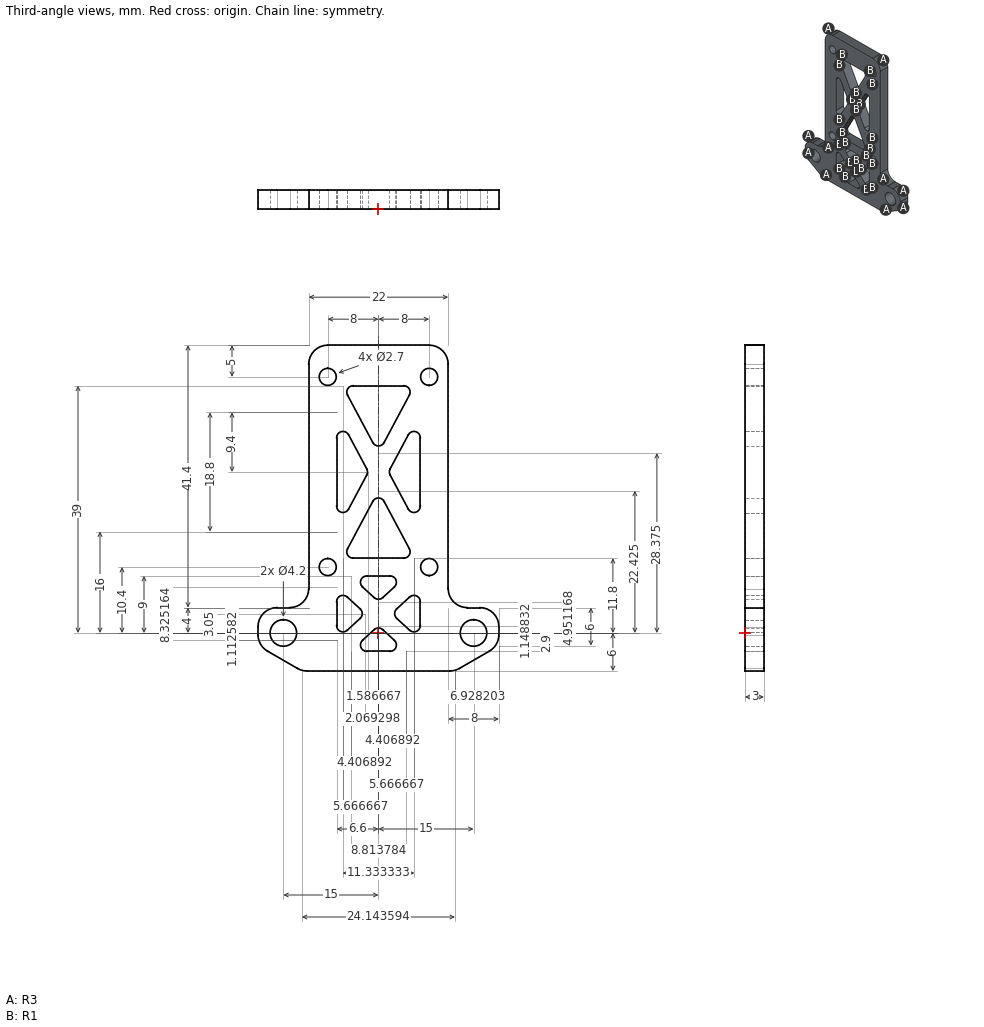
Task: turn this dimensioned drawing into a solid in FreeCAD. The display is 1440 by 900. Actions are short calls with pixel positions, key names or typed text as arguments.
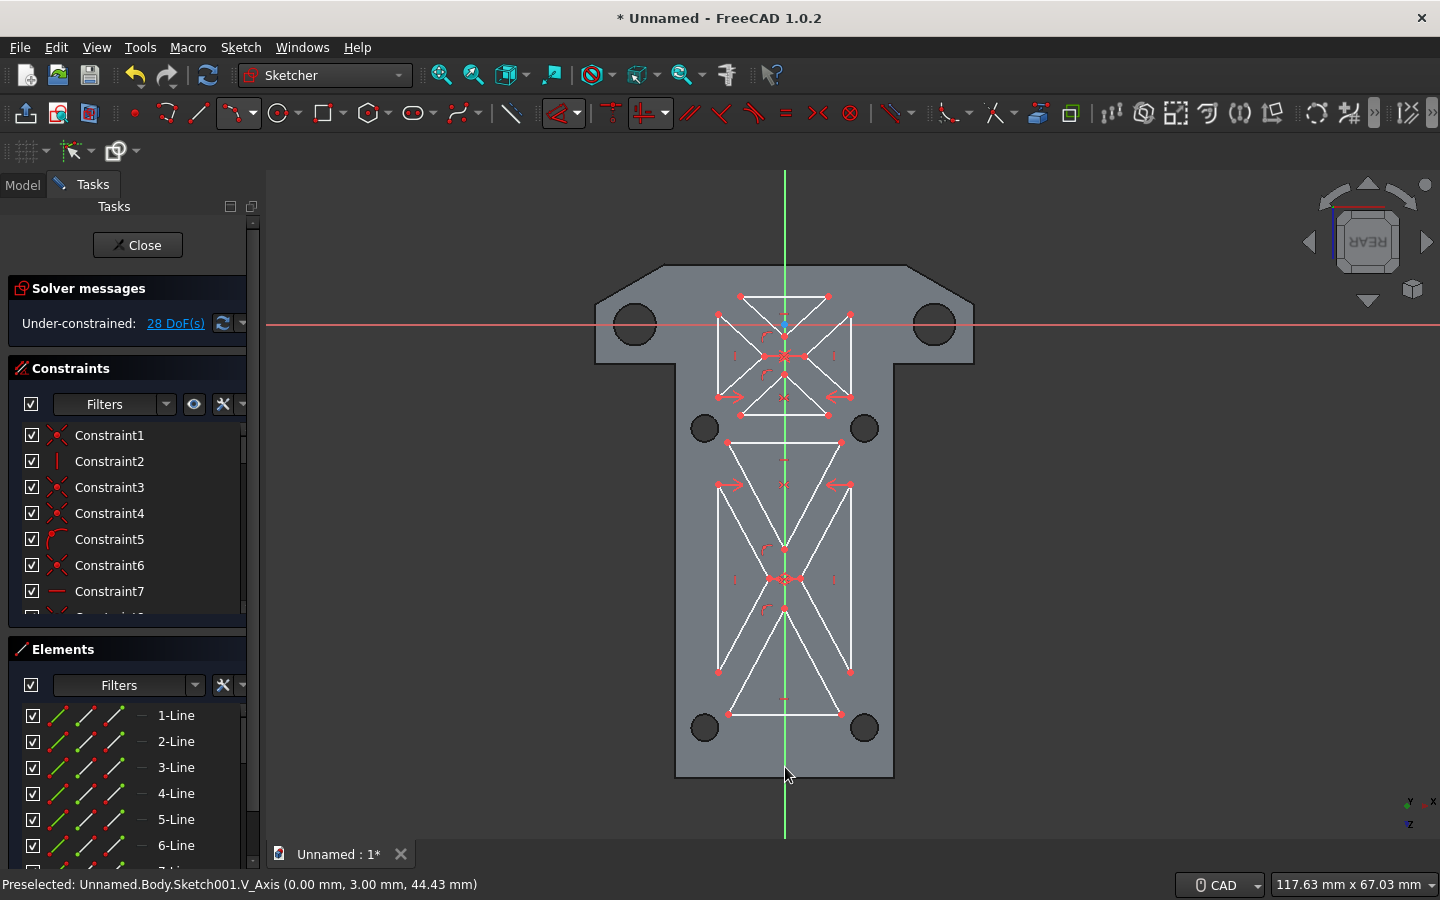
click(558, 114)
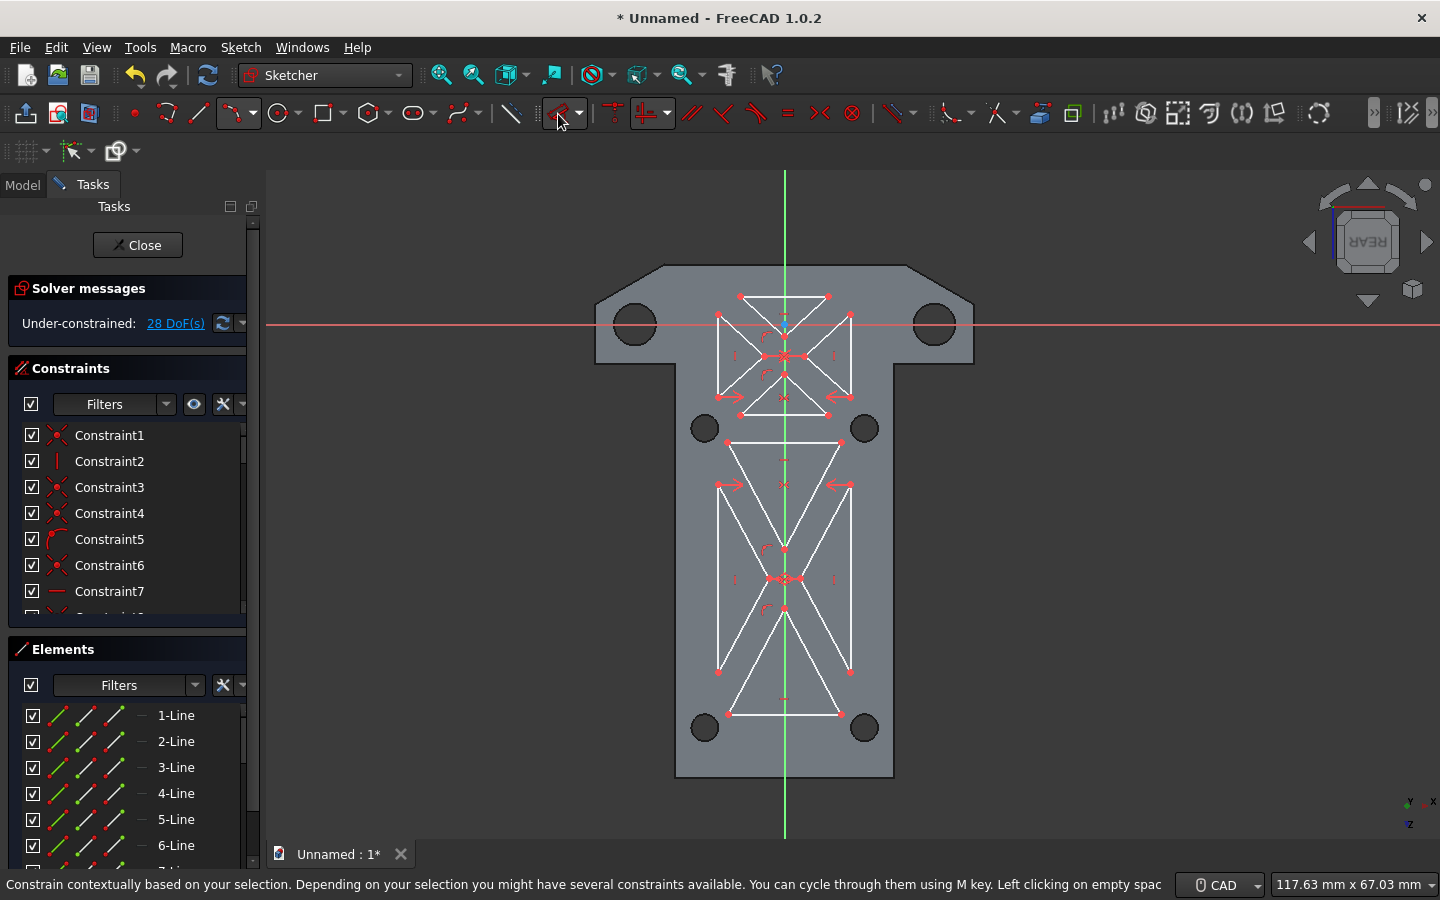
click(741, 415)
click(683, 370)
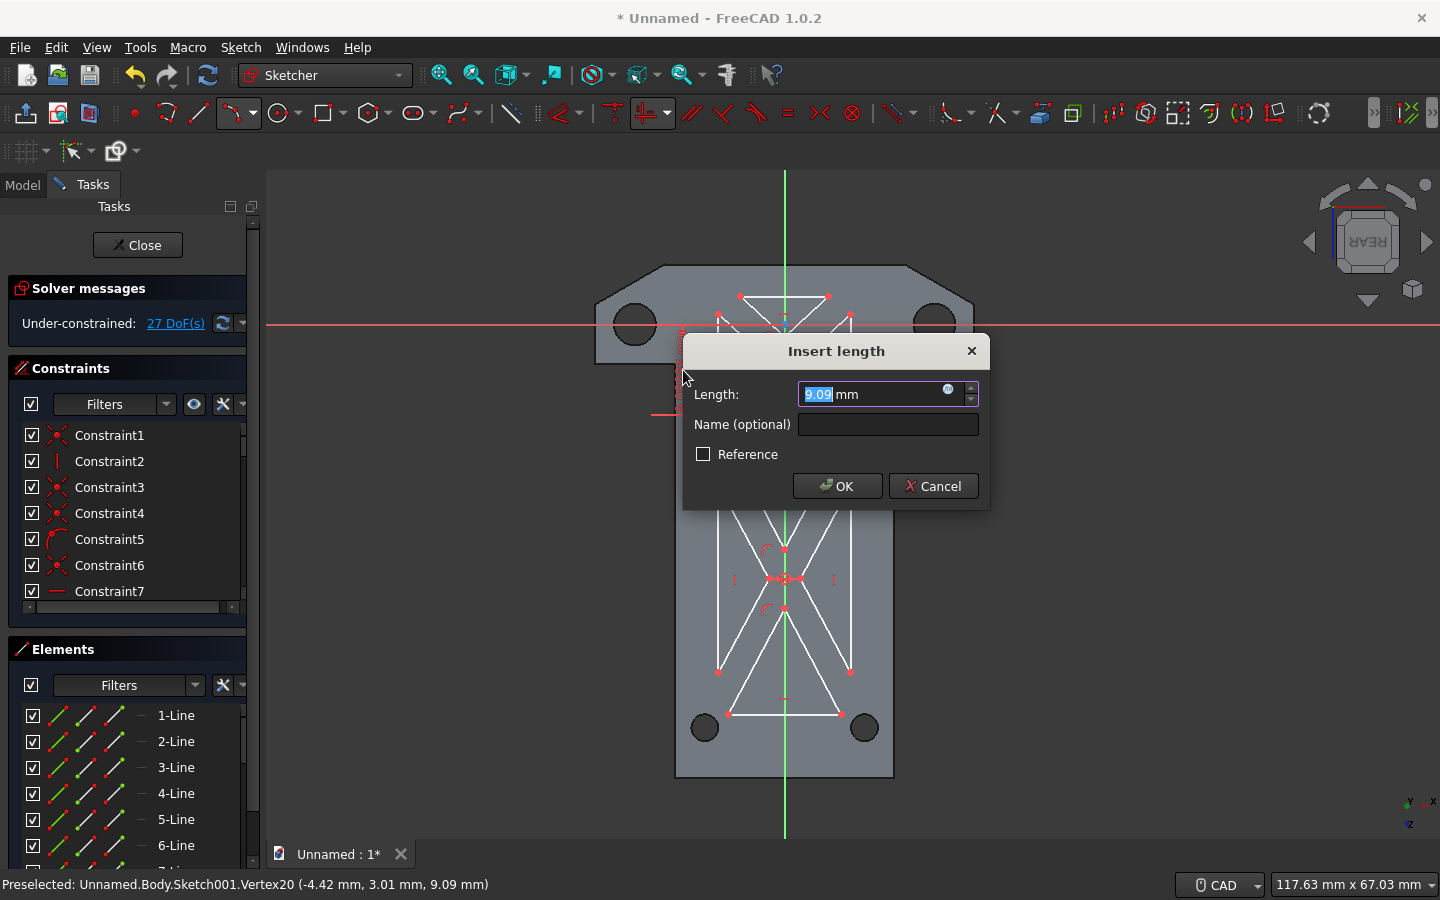
text(9)
key(Return)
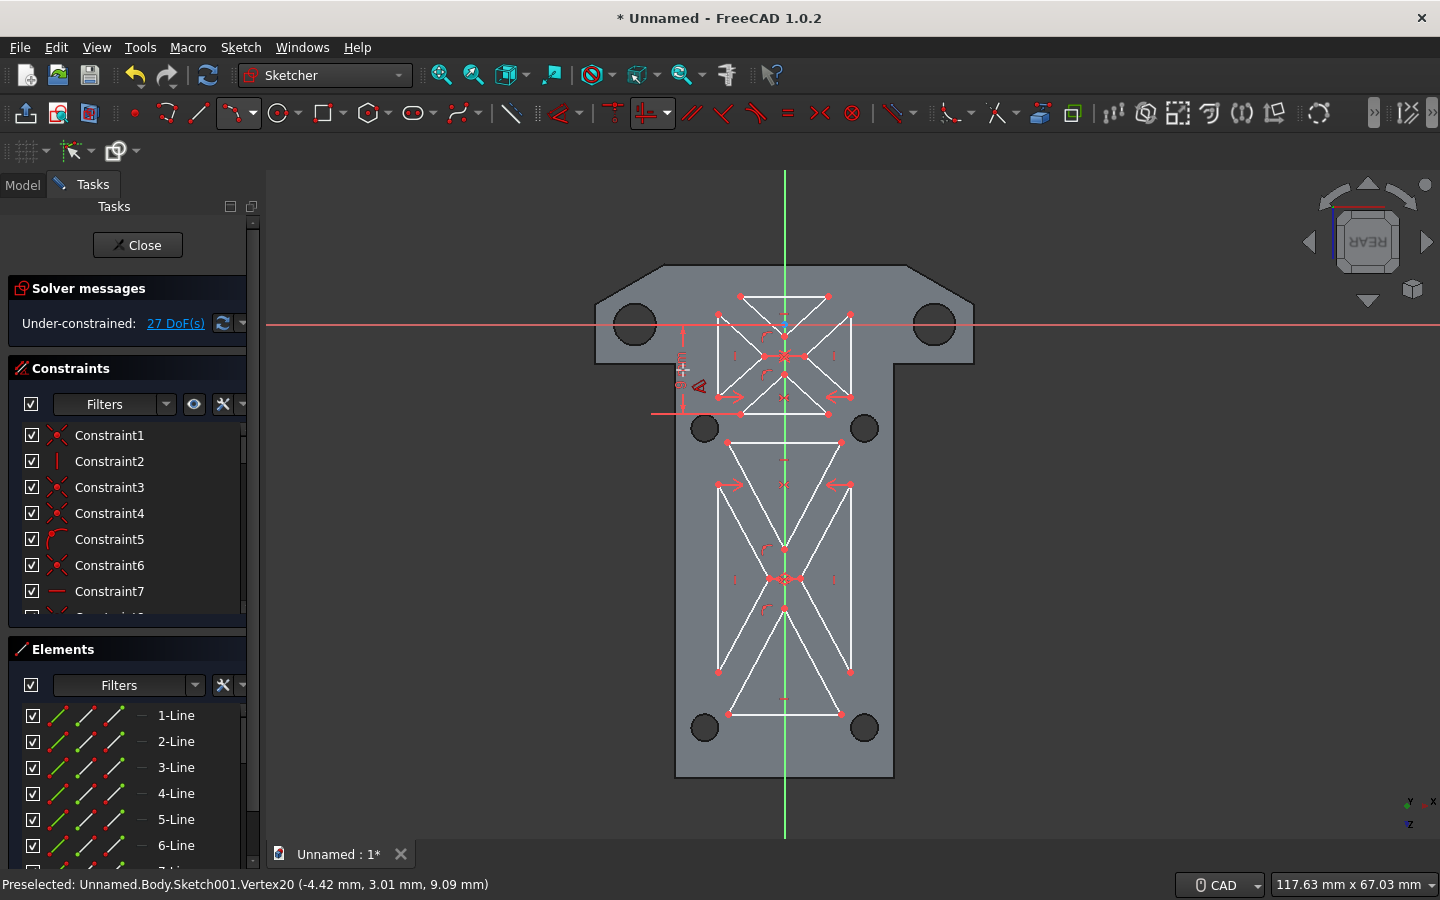
click(718, 485)
click(684, 405)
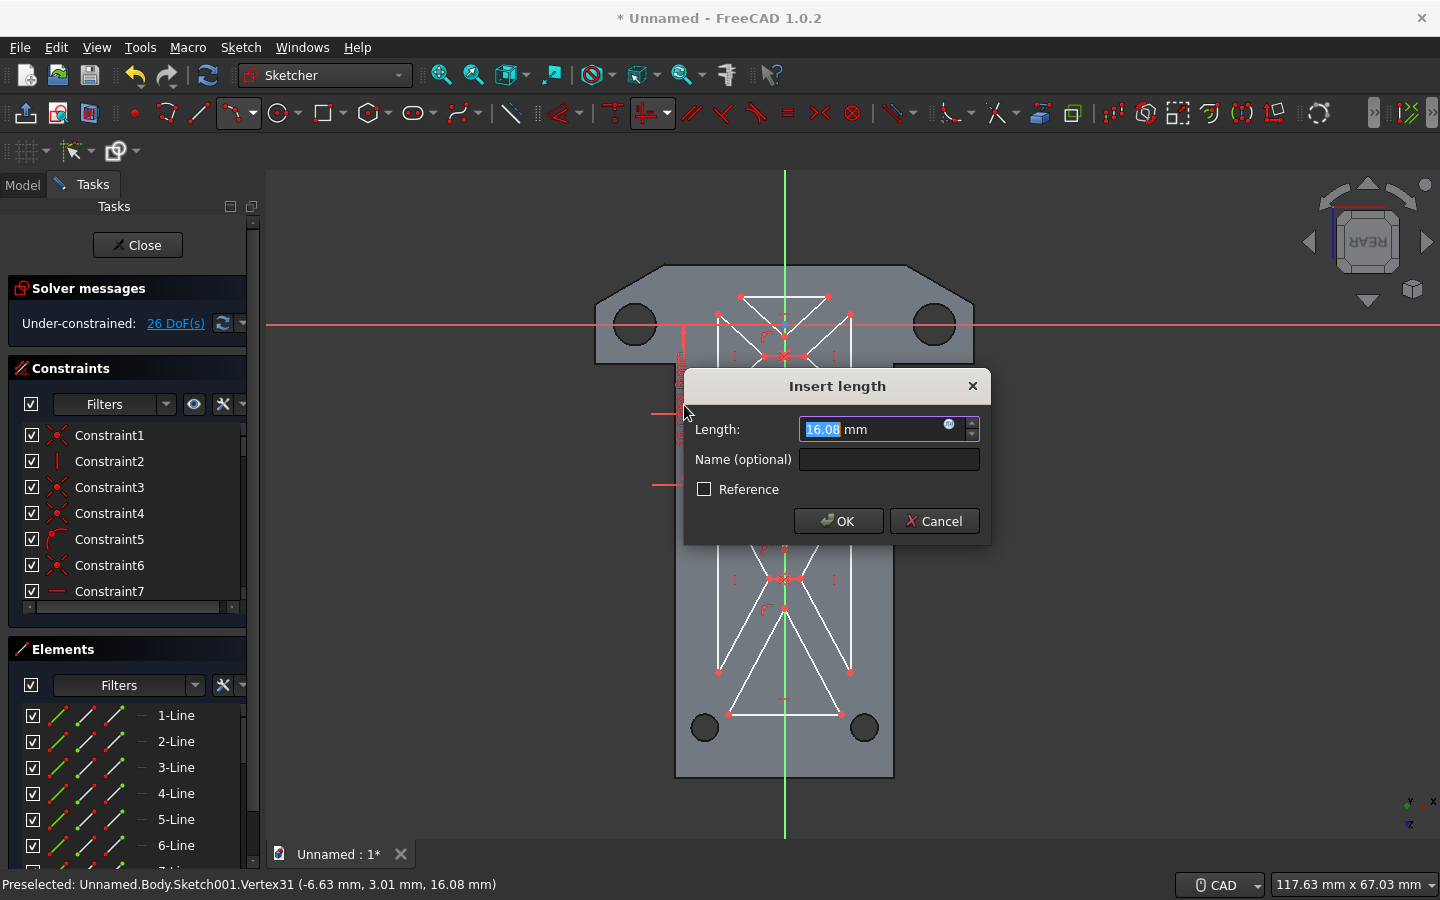
text(16)
key(Return)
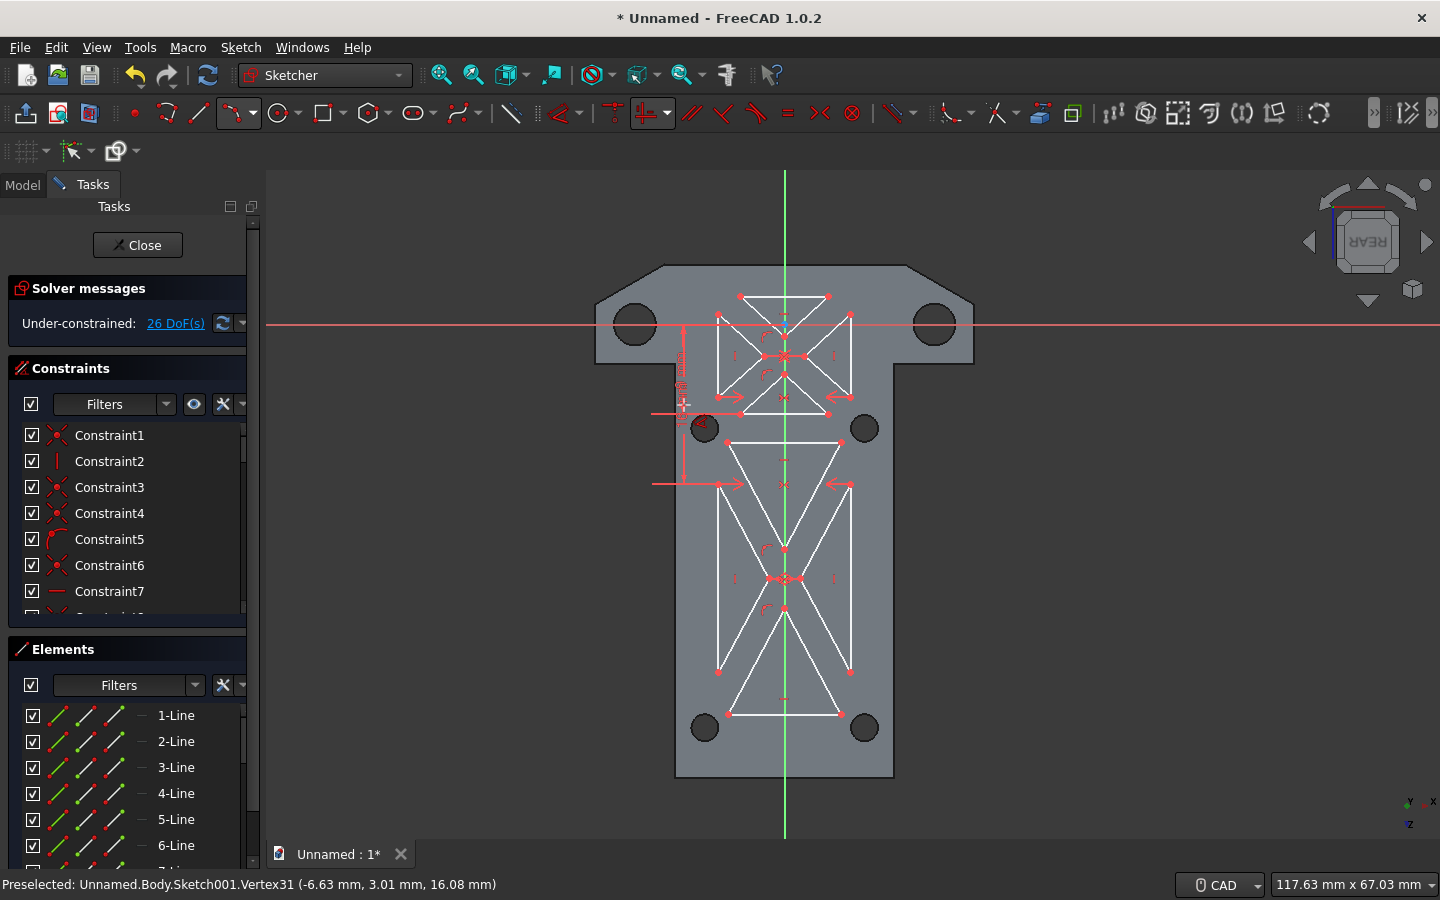
click(728, 715)
click(694, 520)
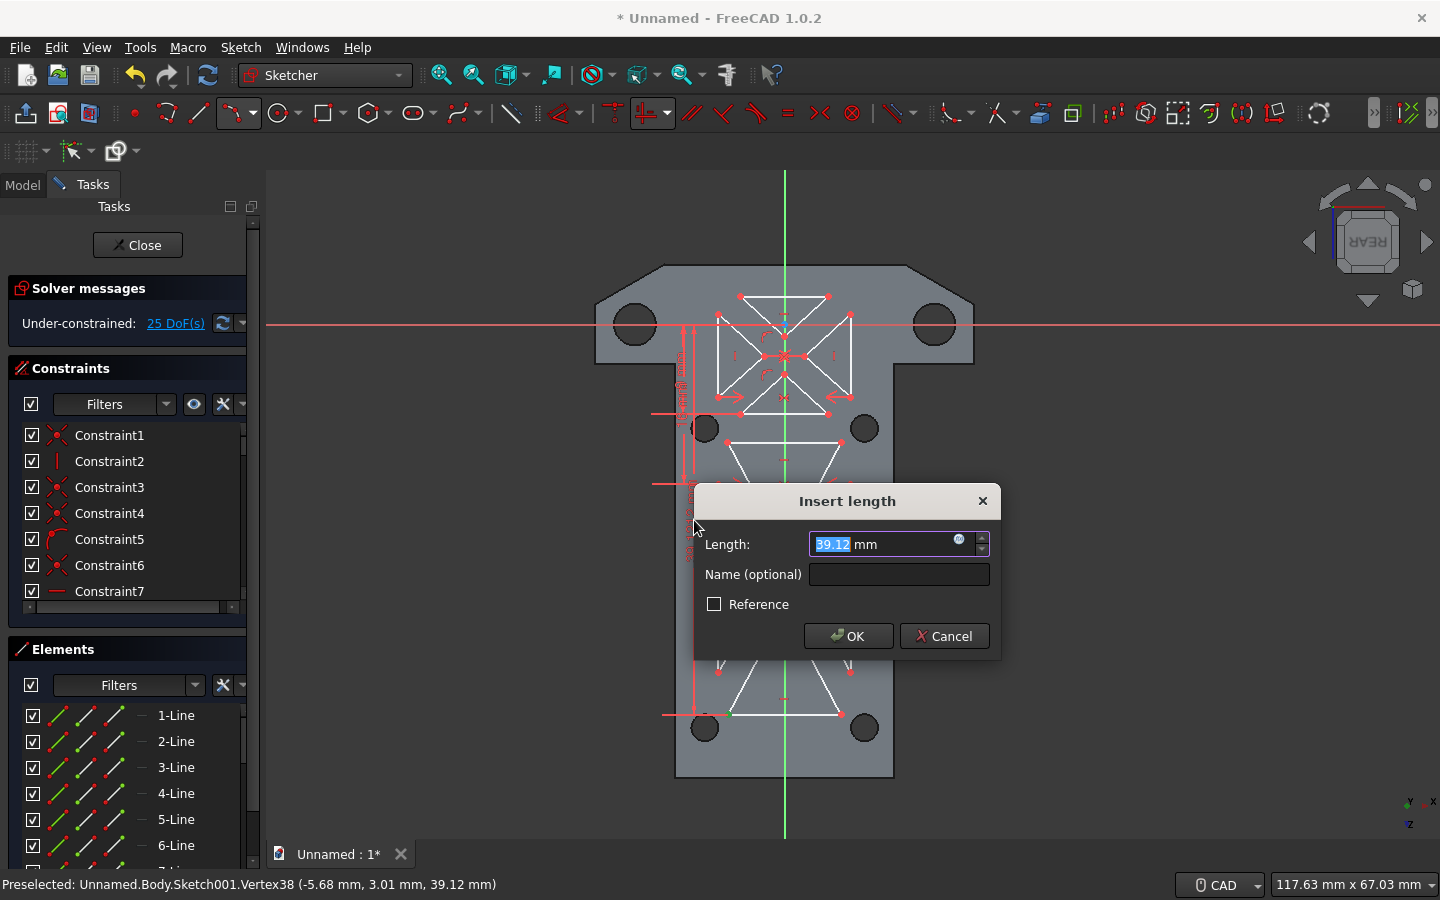
text(39)
key(Return)